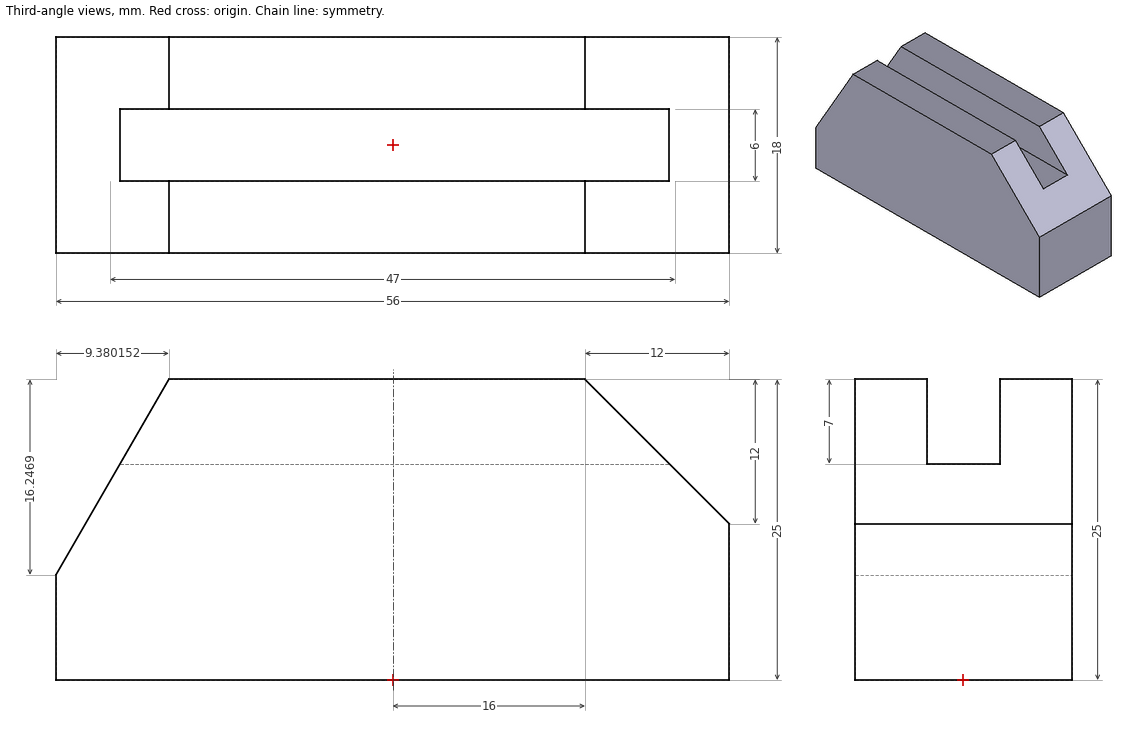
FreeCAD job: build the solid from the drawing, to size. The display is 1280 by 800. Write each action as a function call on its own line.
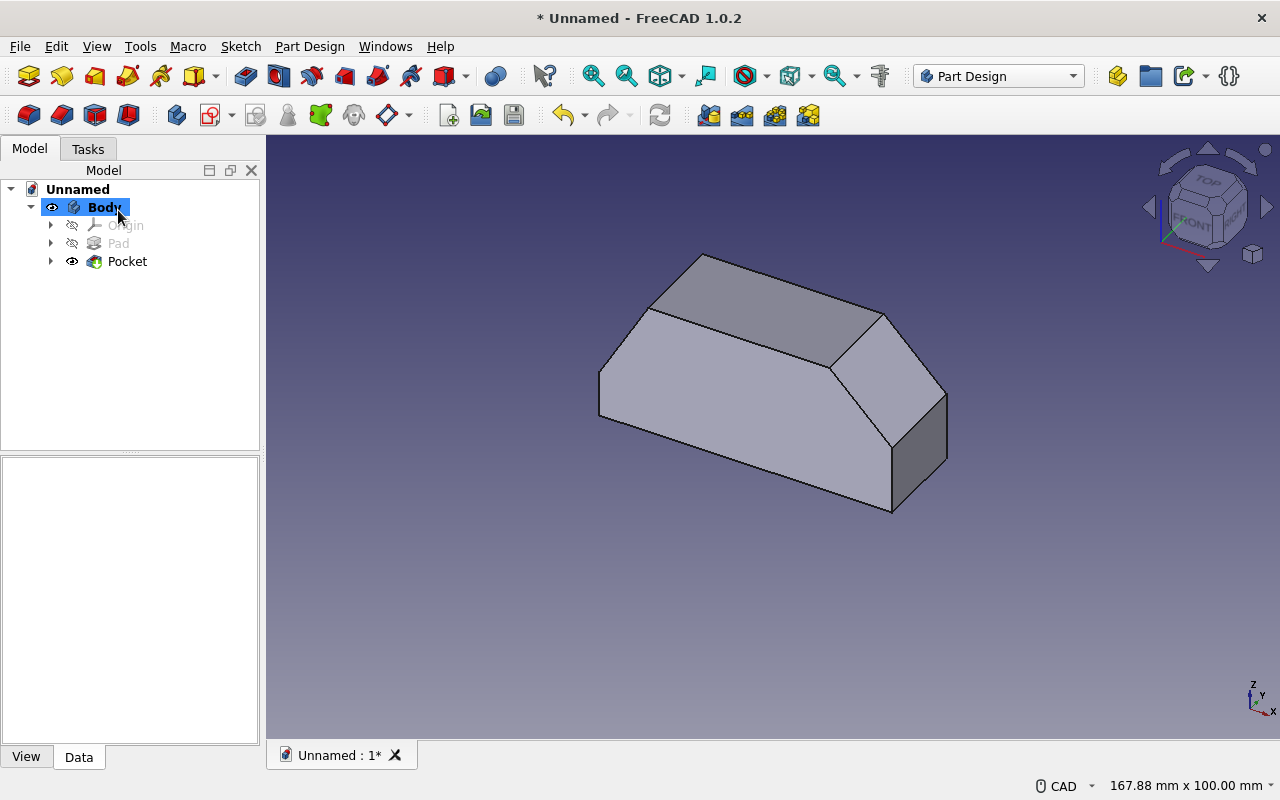
click(792, 319)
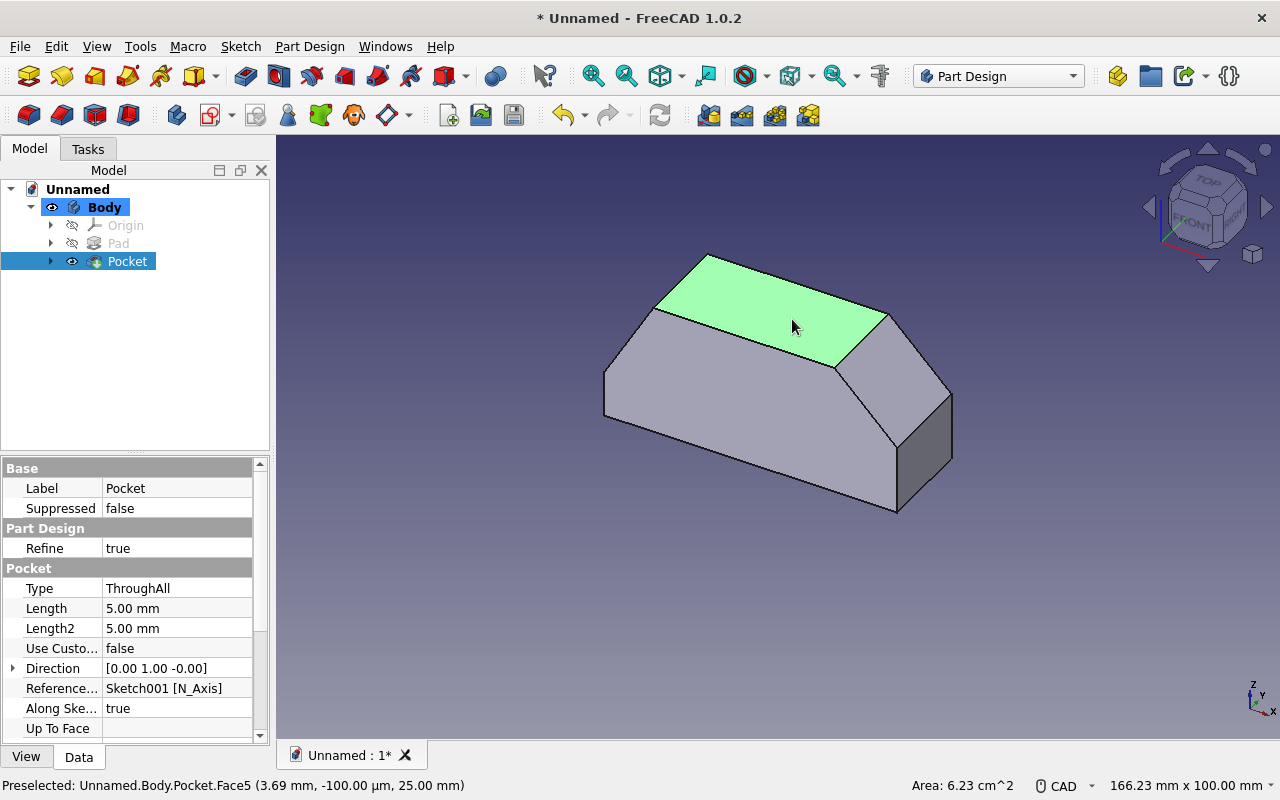
click(210, 116)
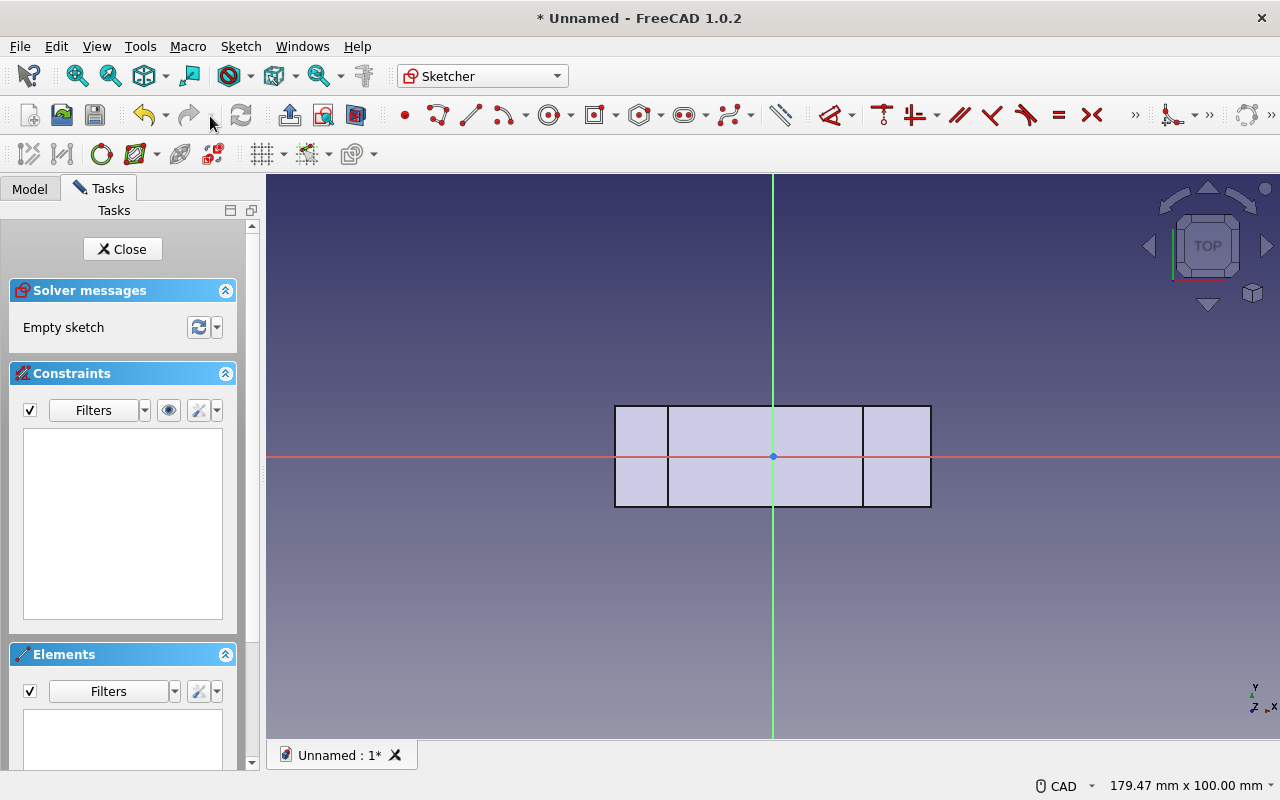
scroll(829, 456, up, 4)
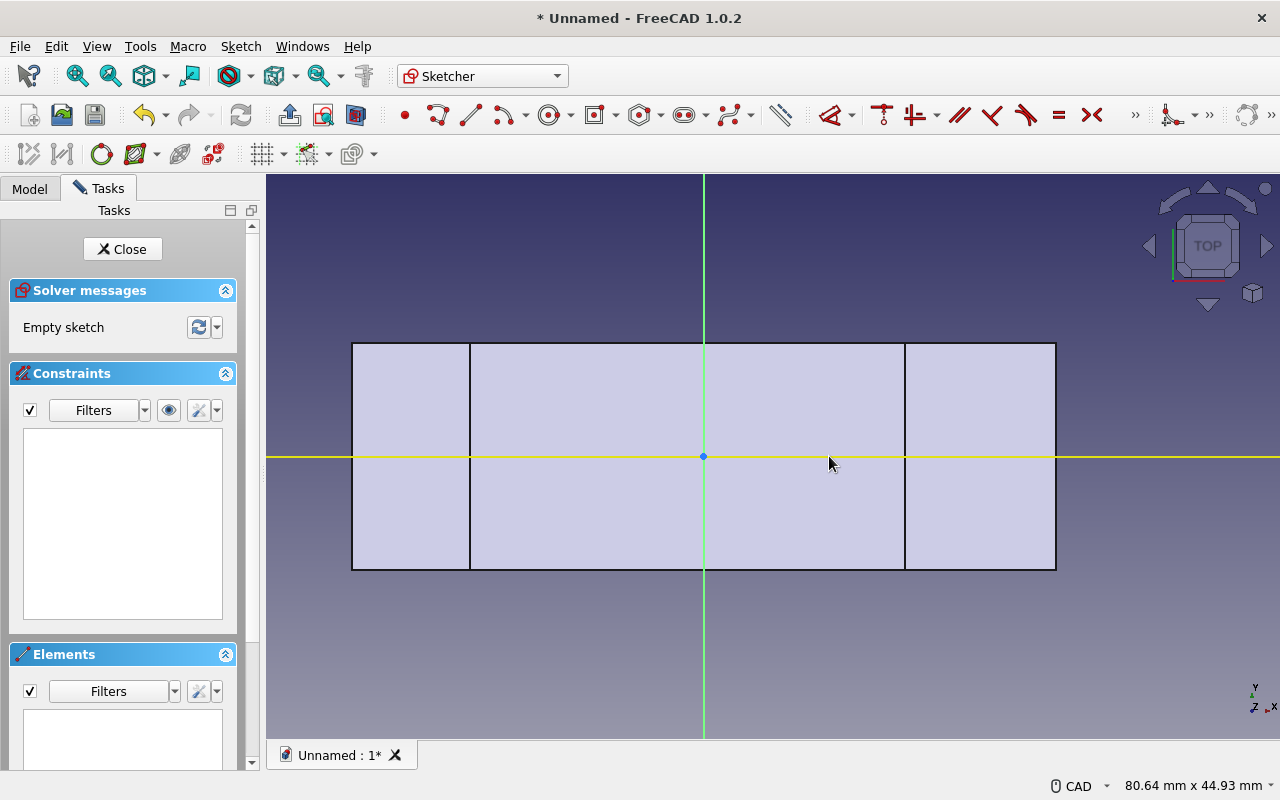
key(g)
key(v)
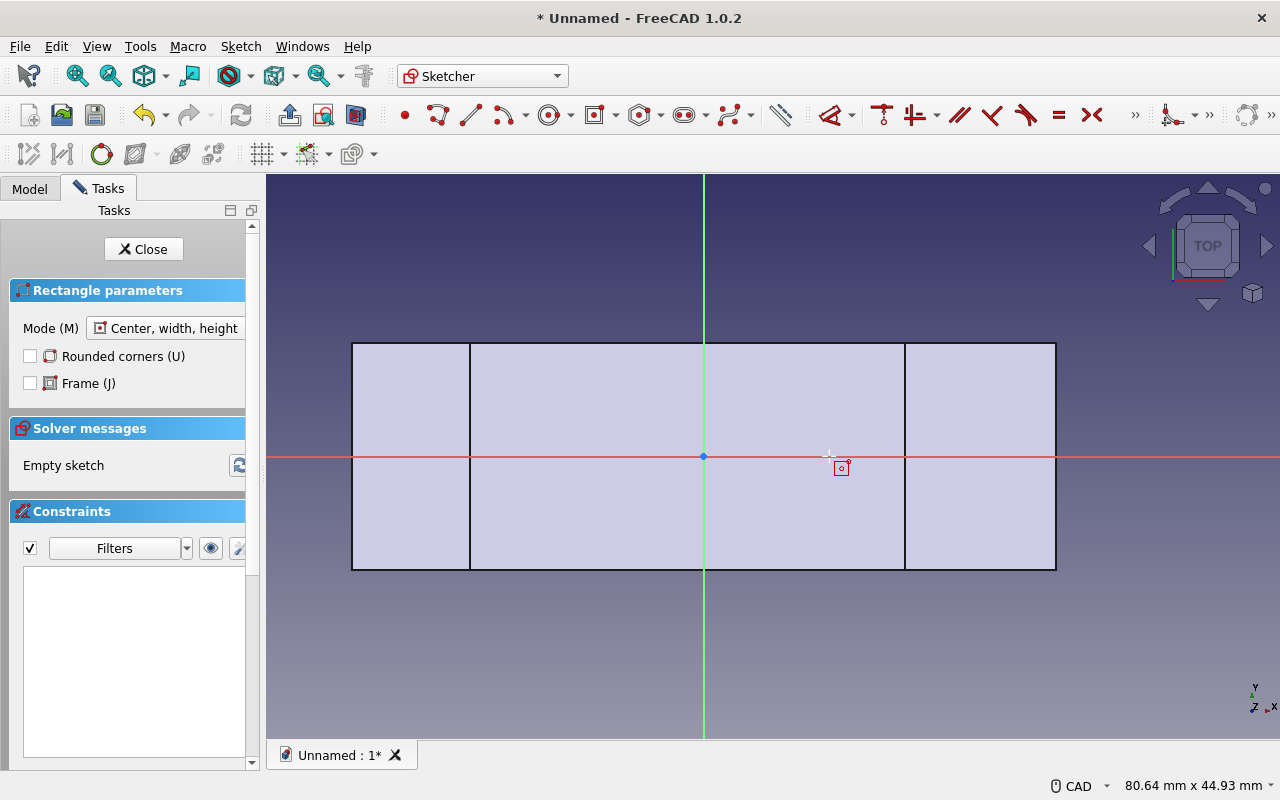
click(704, 456)
move(999, 419)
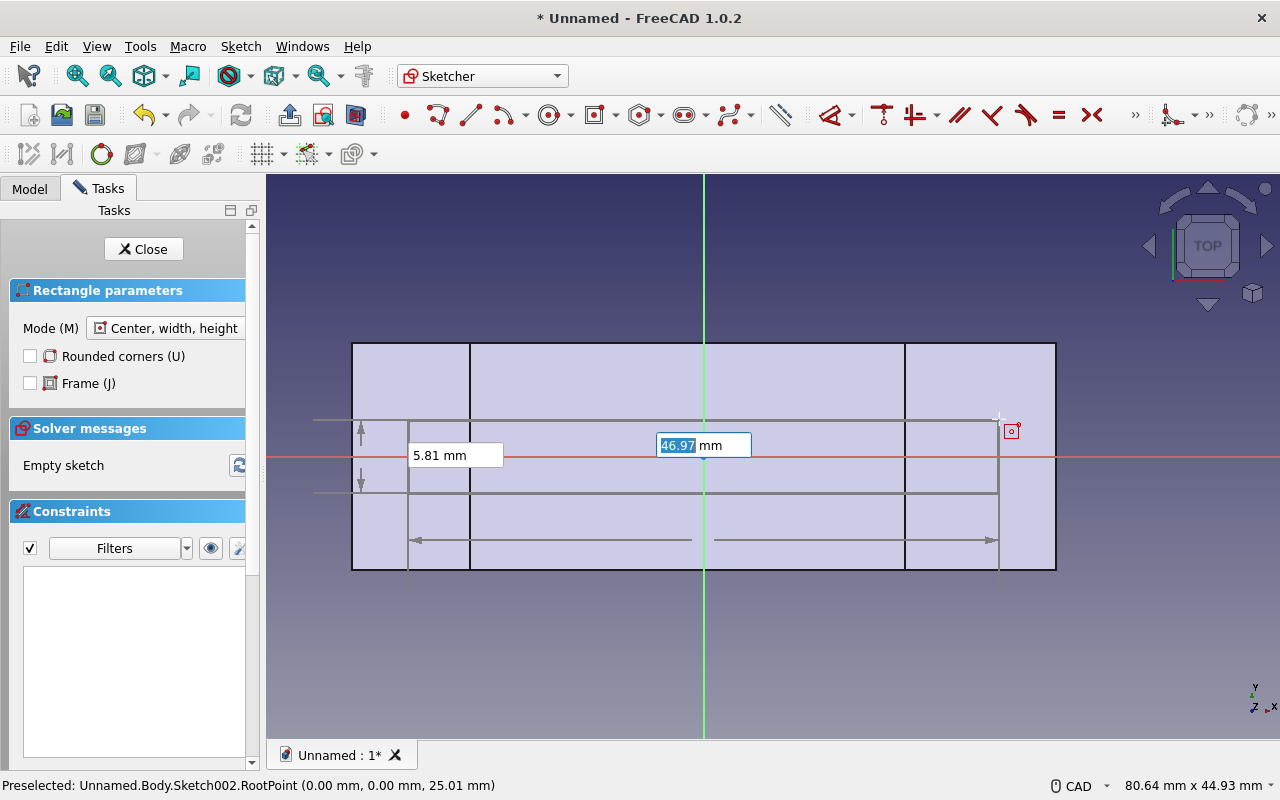
text(47)
key(Tab)
text(6)
key(Return)
key(Escape)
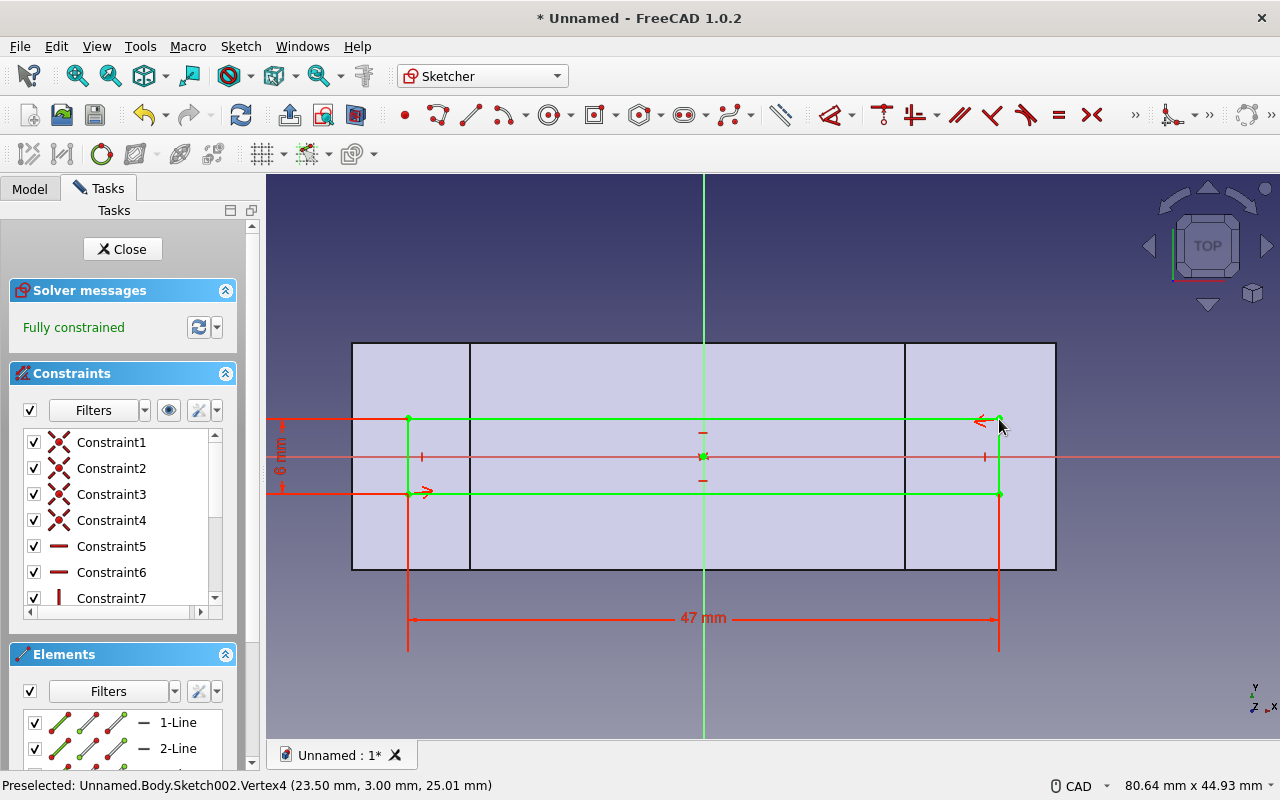
click(123, 249)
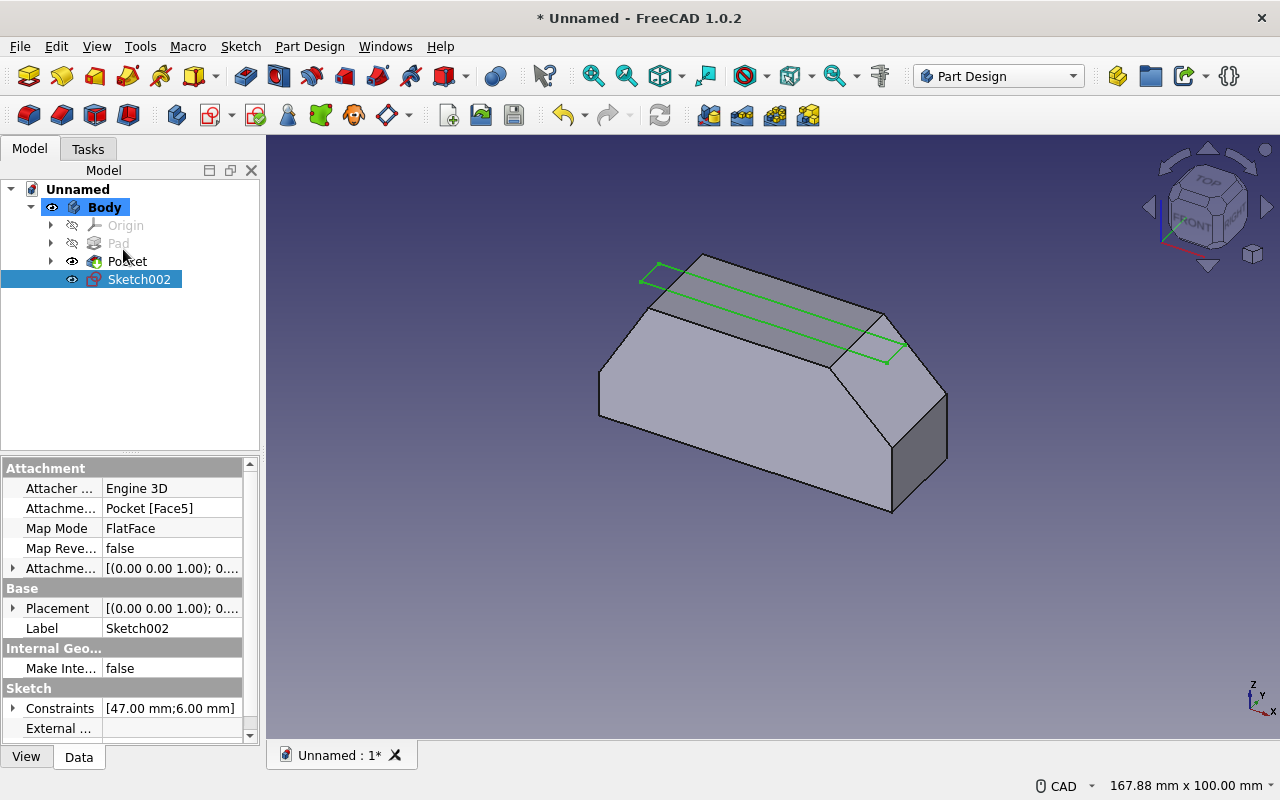
click(246, 76)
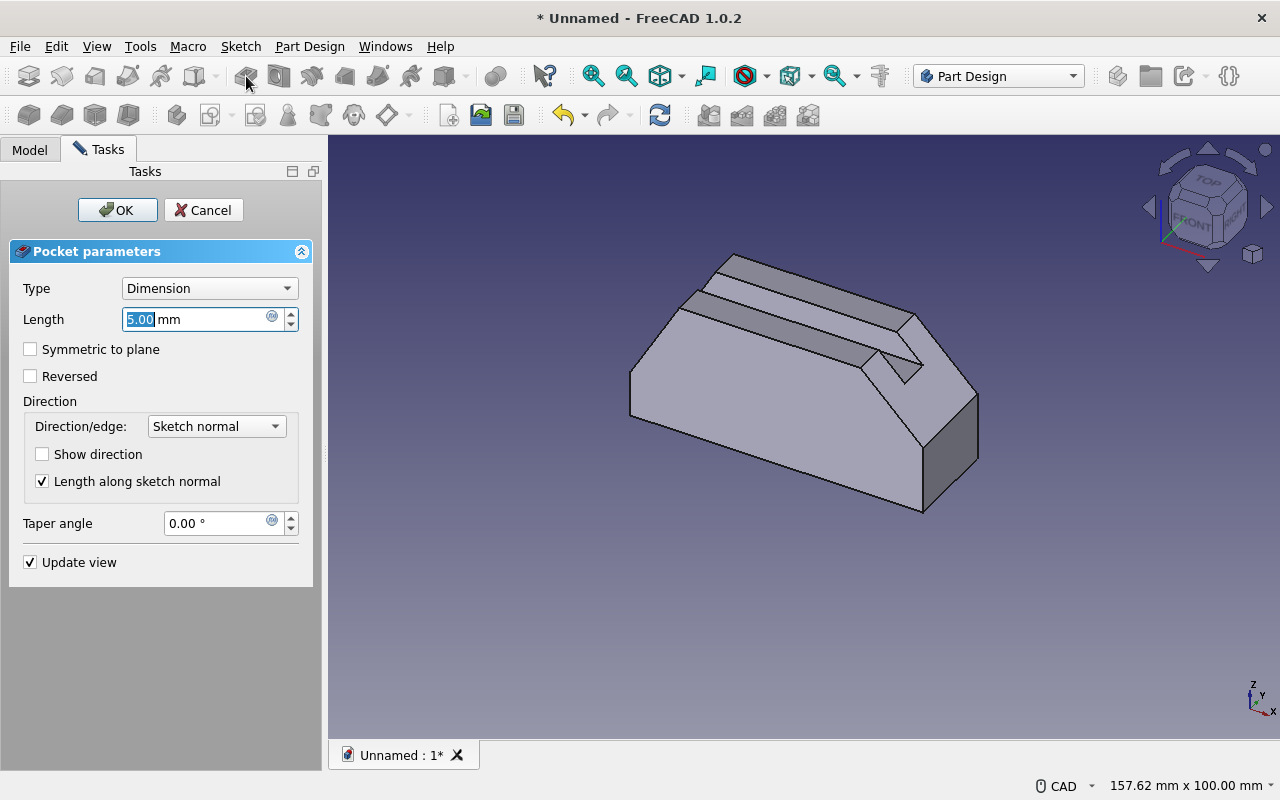
text(7)
key(Tab)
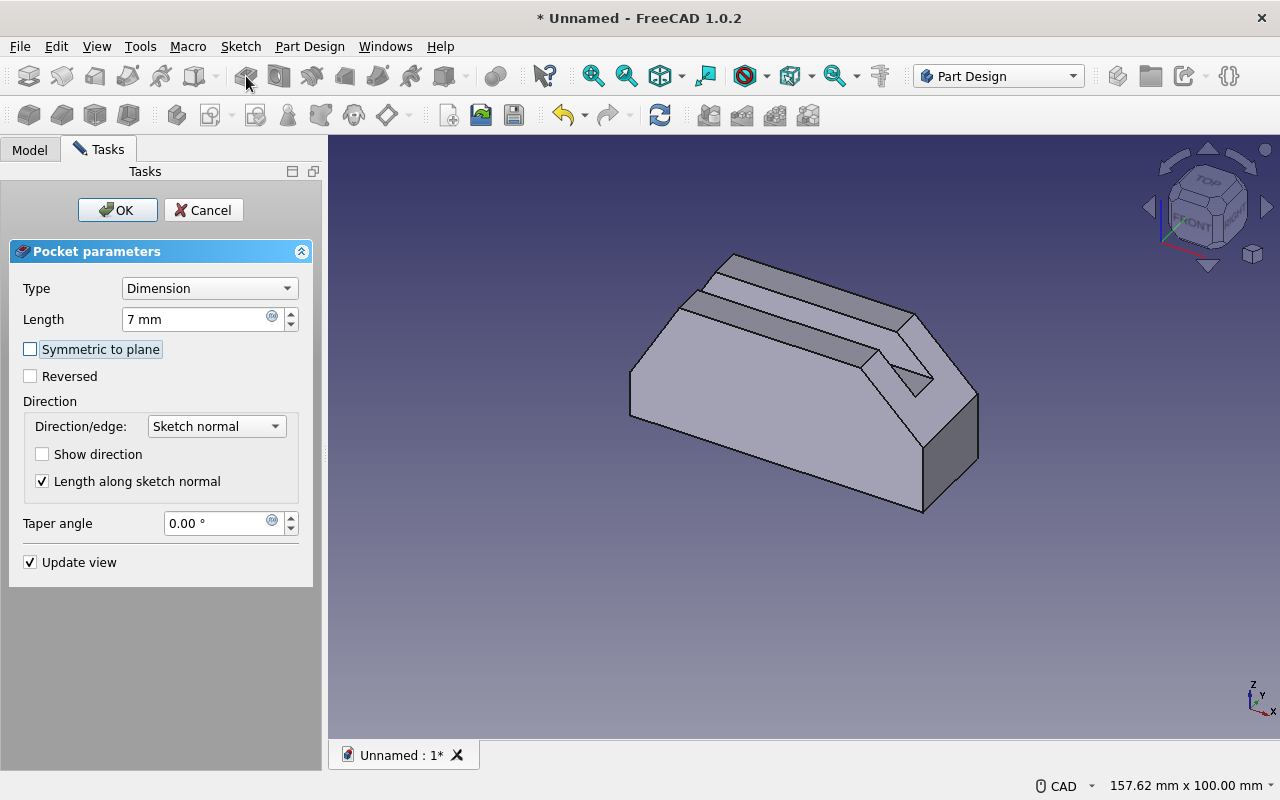
click(118, 210)